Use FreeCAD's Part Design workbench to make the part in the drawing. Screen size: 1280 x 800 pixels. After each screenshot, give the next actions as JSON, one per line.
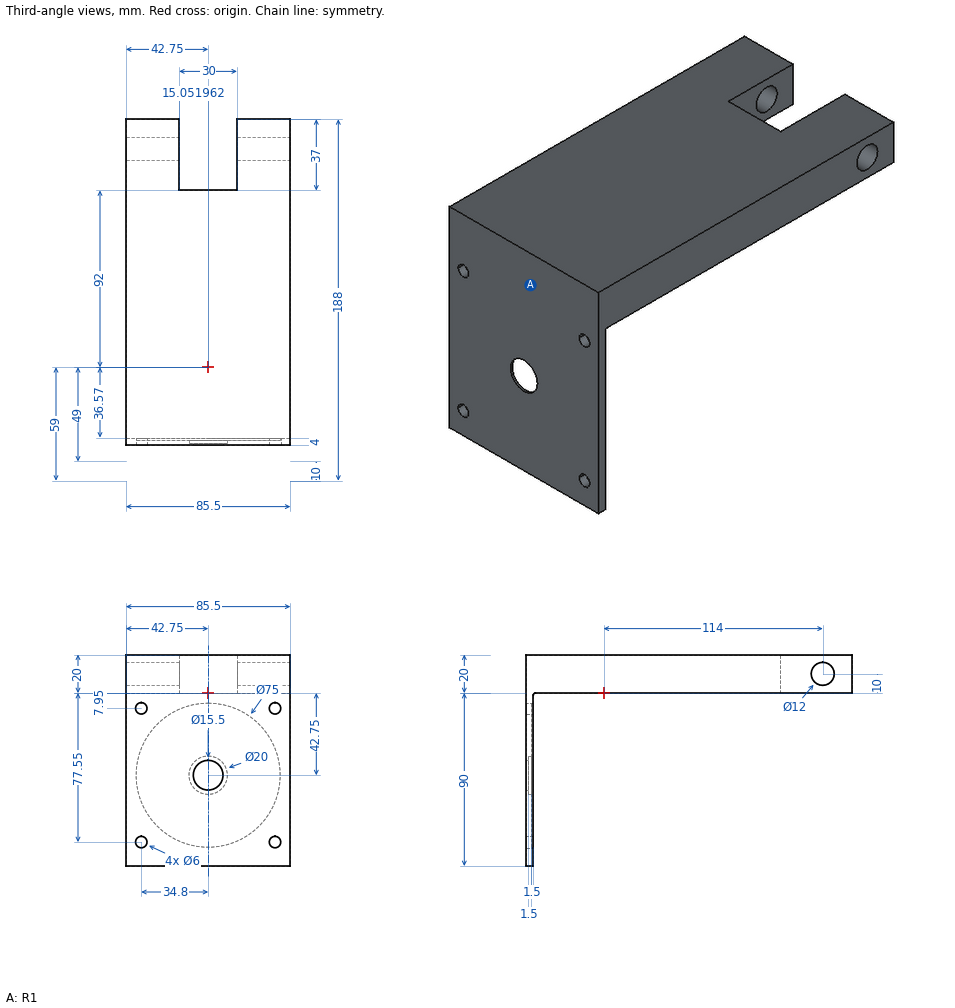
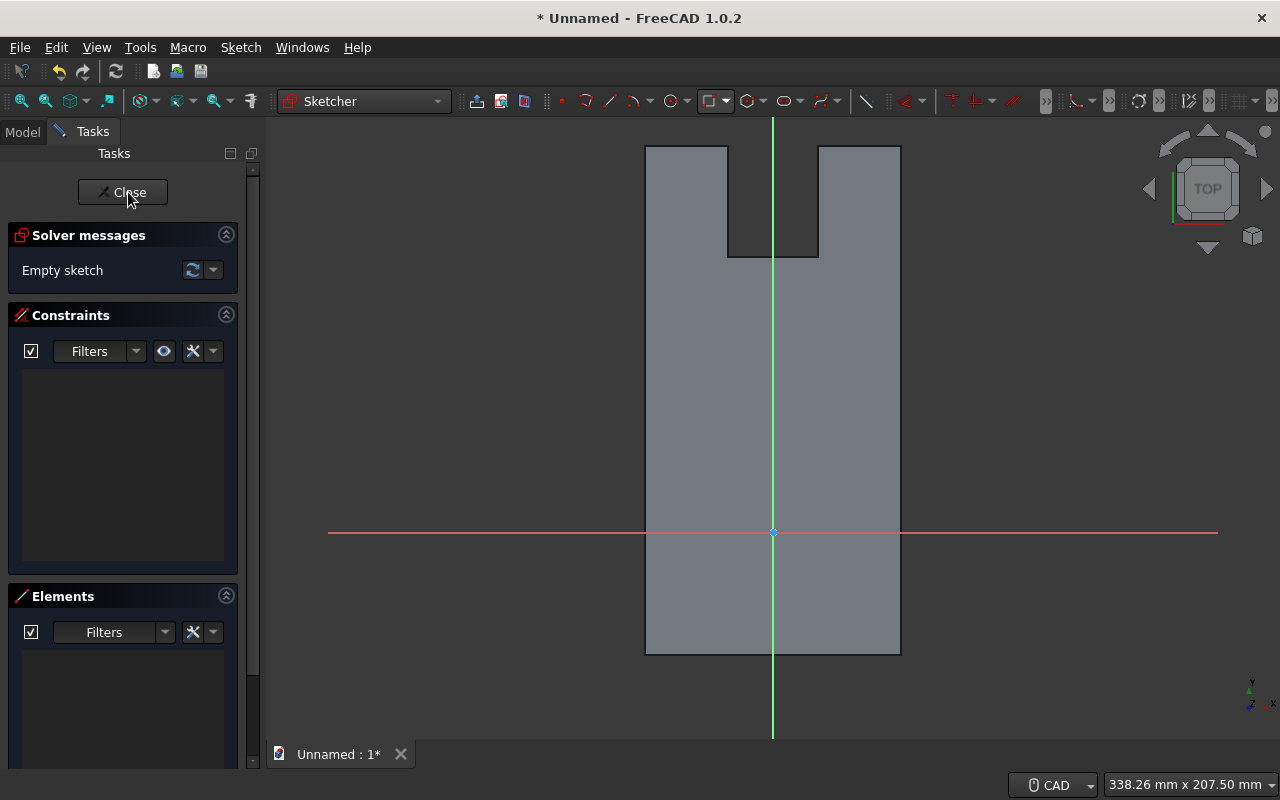
{"action": "scroll", "coordinate": [829, 711], "scroll_direction": "up", "scroll_amount": 4}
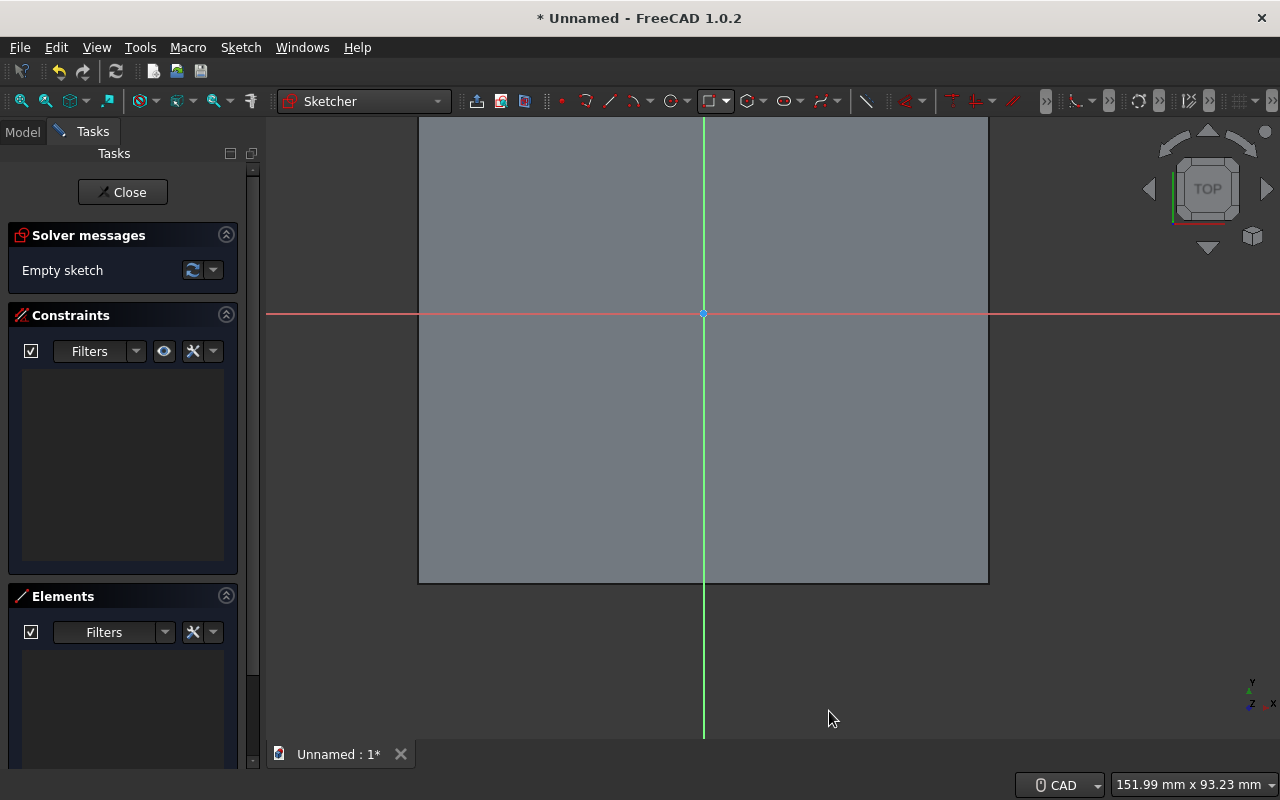
{"action": "key", "text": "g r"}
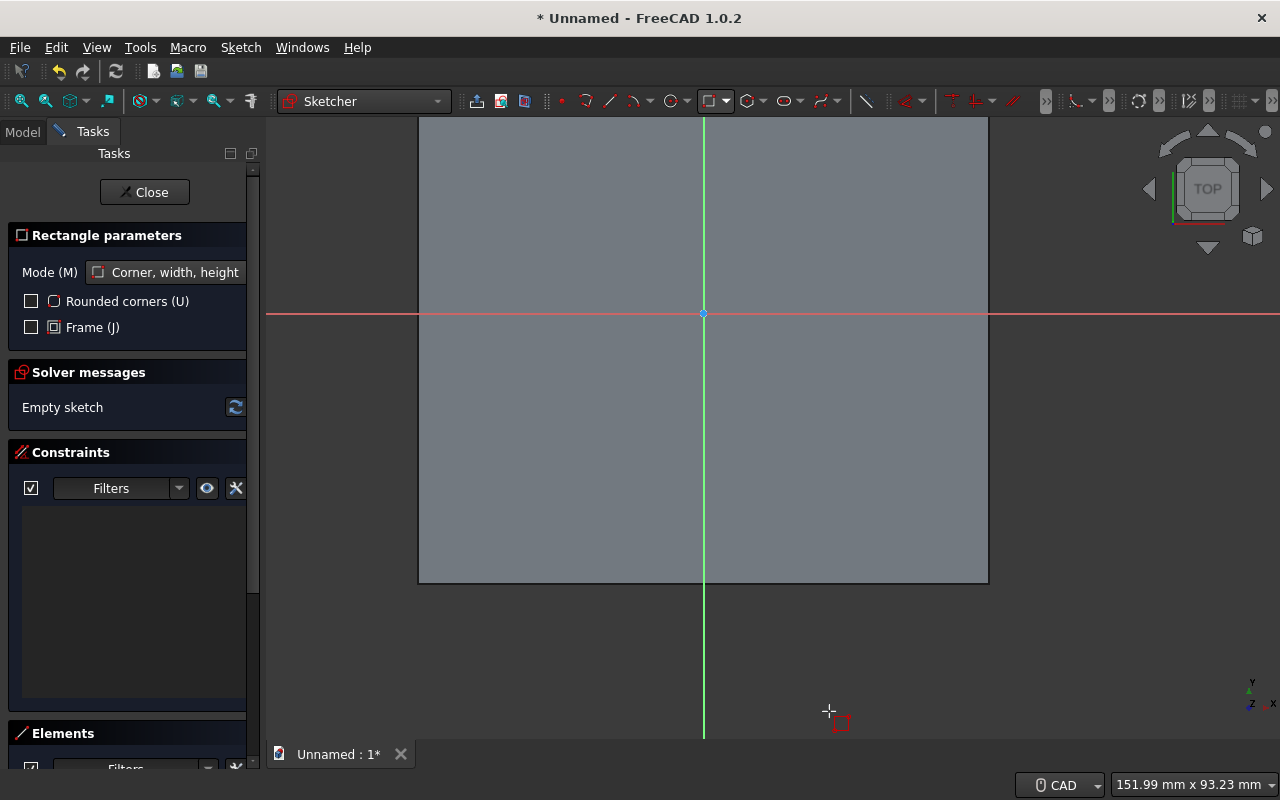
{"action": "left_click", "coordinate": [418, 557]}
{"action": "mouse_move", "coordinate": [989, 584]}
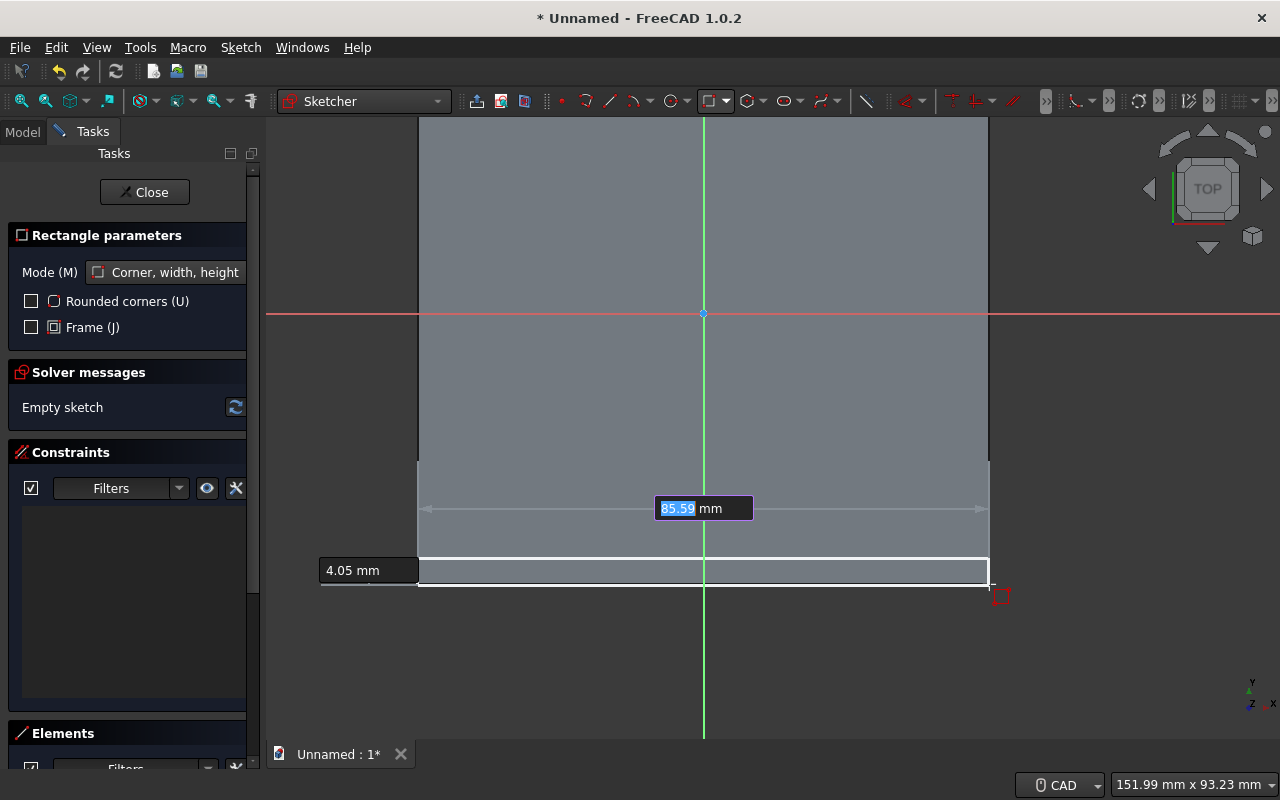
{"action": "type", "text": "85.5"}
{"action": "key", "text": "Tab"}
{"action": "type", "text": "4"}
{"action": "key", "text": "Return"}
{"action": "key", "text": "Escape"}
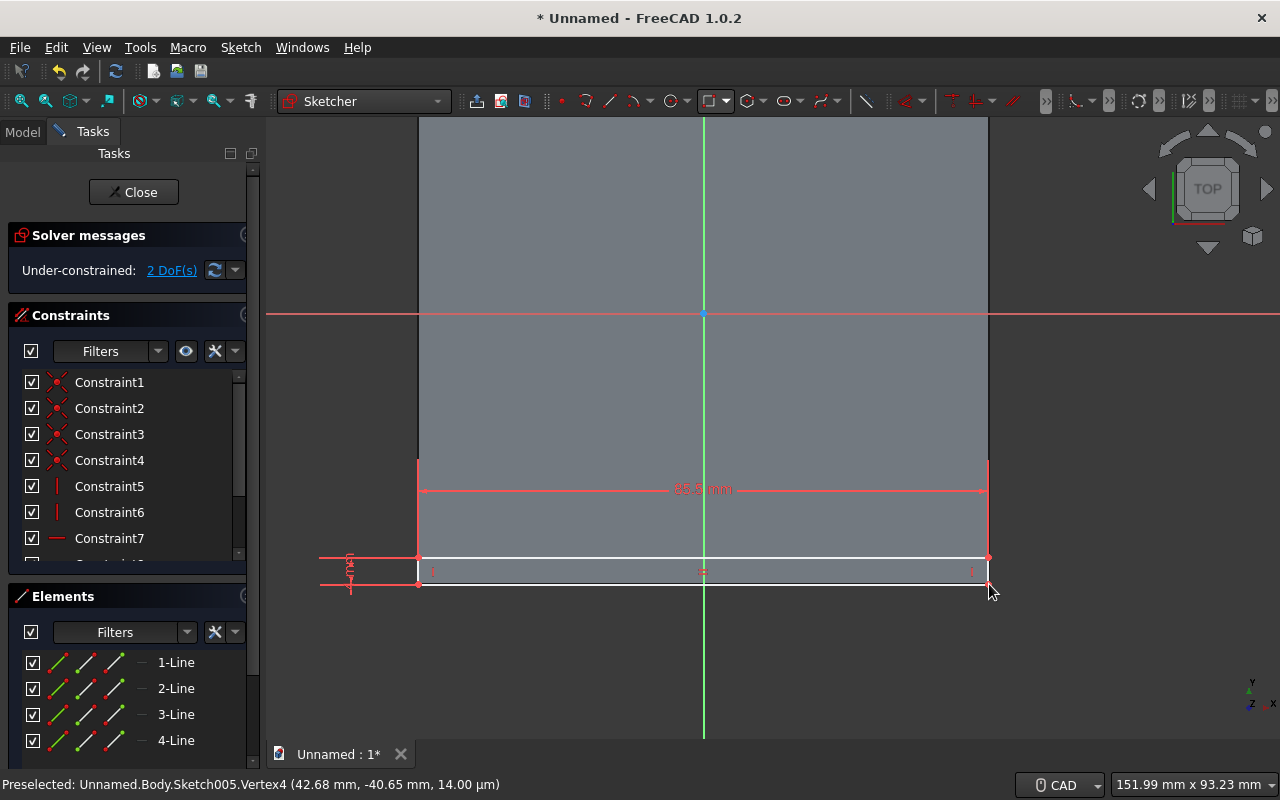
{"action": "key", "text": "d"}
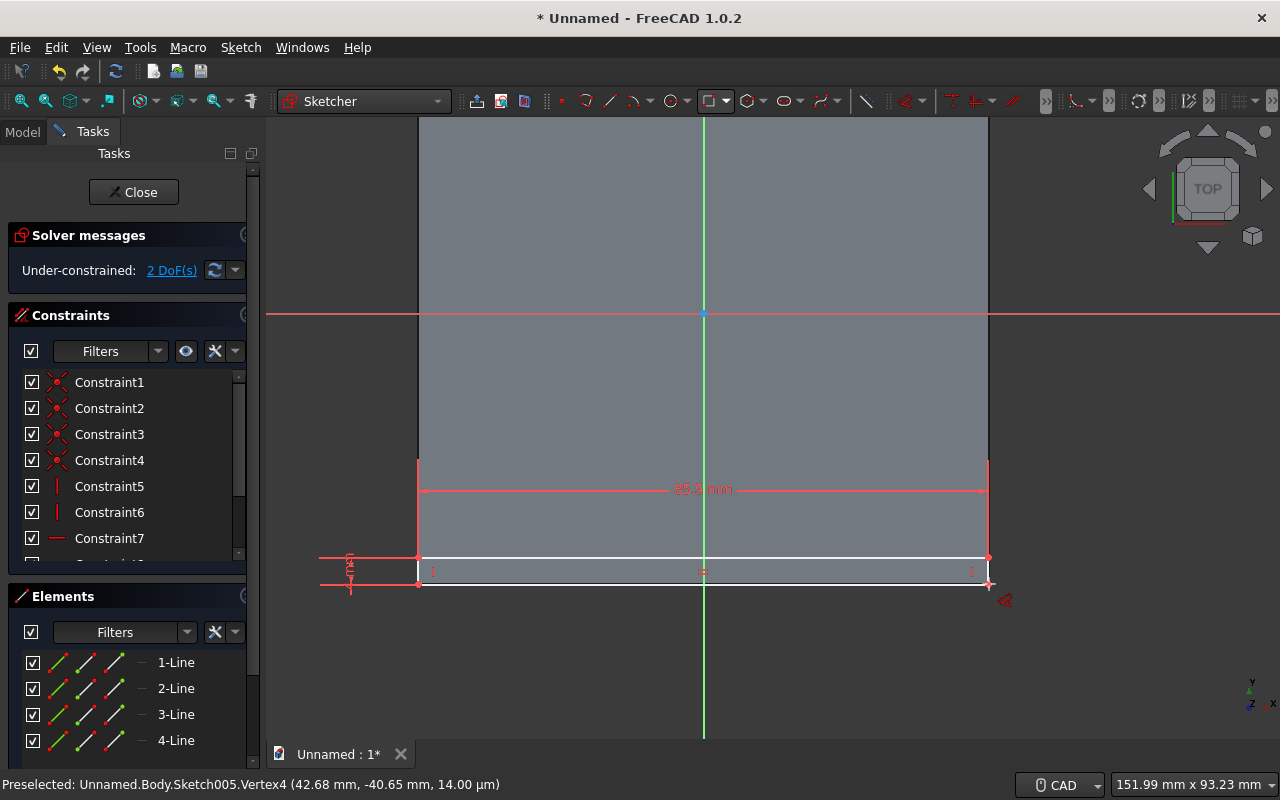
{"action": "left_click", "coordinate": [418, 558]}
{"action": "left_click", "coordinate": [561, 279]}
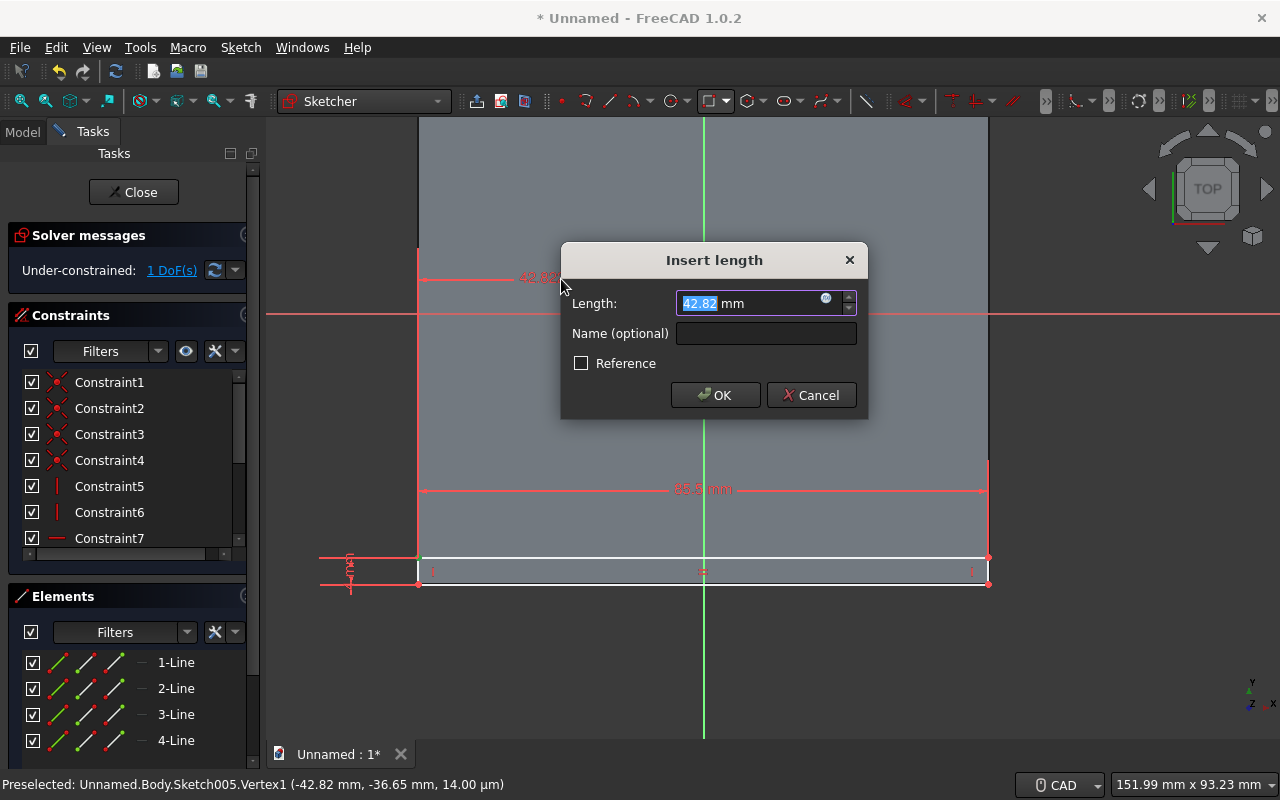
{"action": "type", "text": "42.75"}
{"action": "key", "text": "Return"}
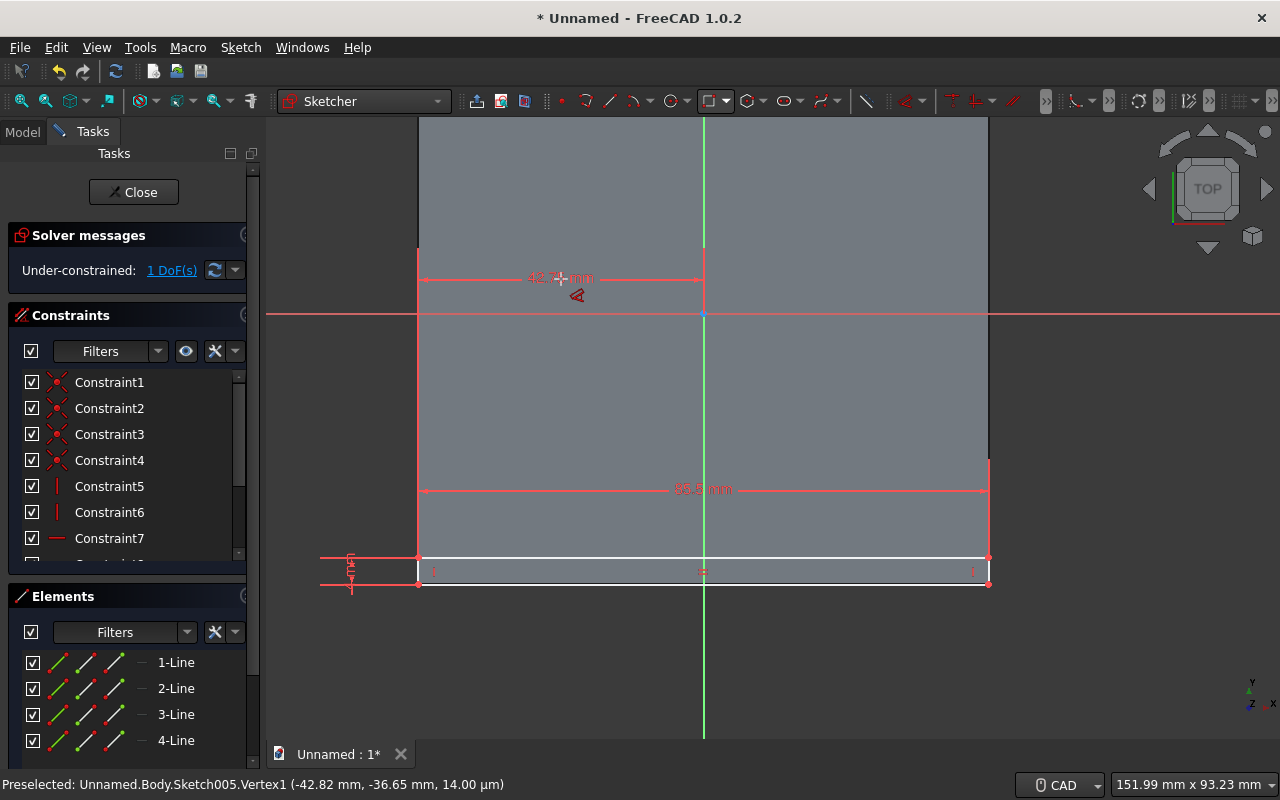
{"action": "left_click", "coordinate": [418, 558]}
{"action": "left_click", "coordinate": [384, 436]}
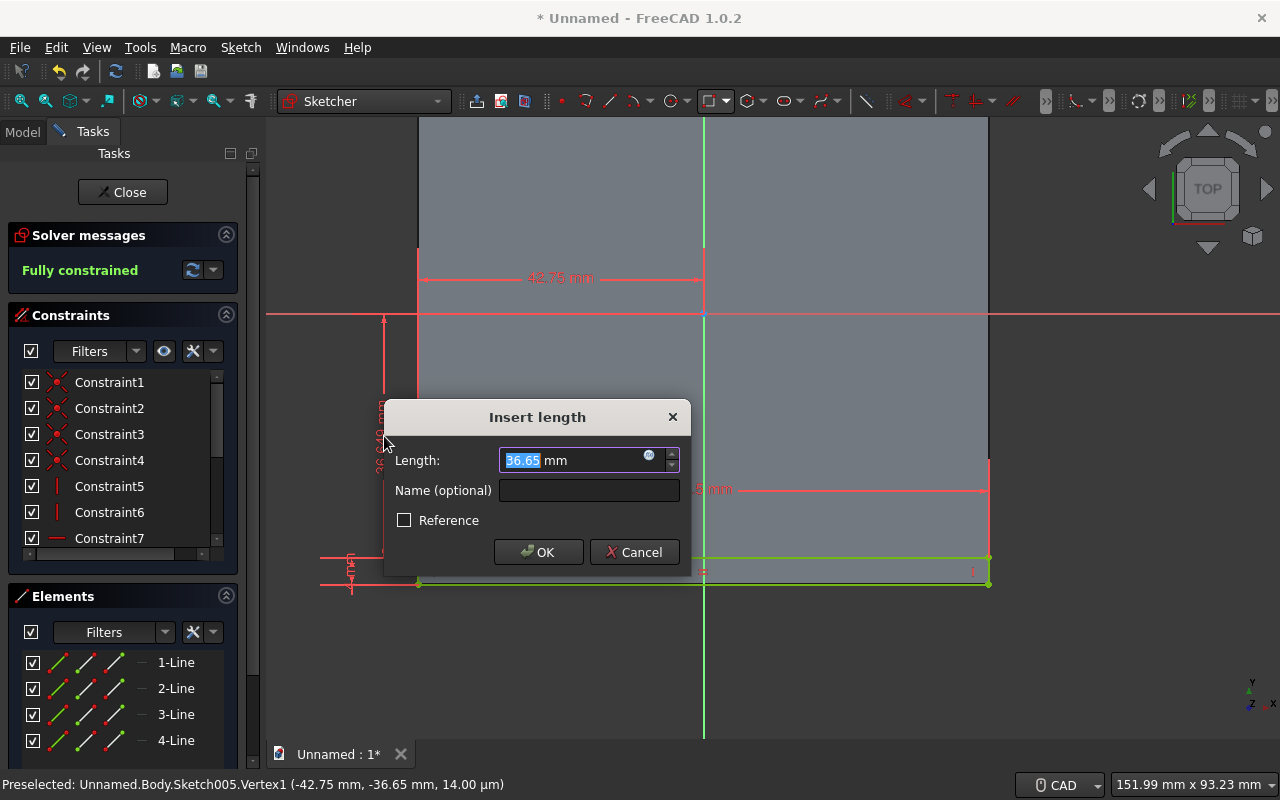
{"action": "type", "text": "36.57"}
{"action": "key", "text": "Return"}
{"action": "key", "text": "Escape"}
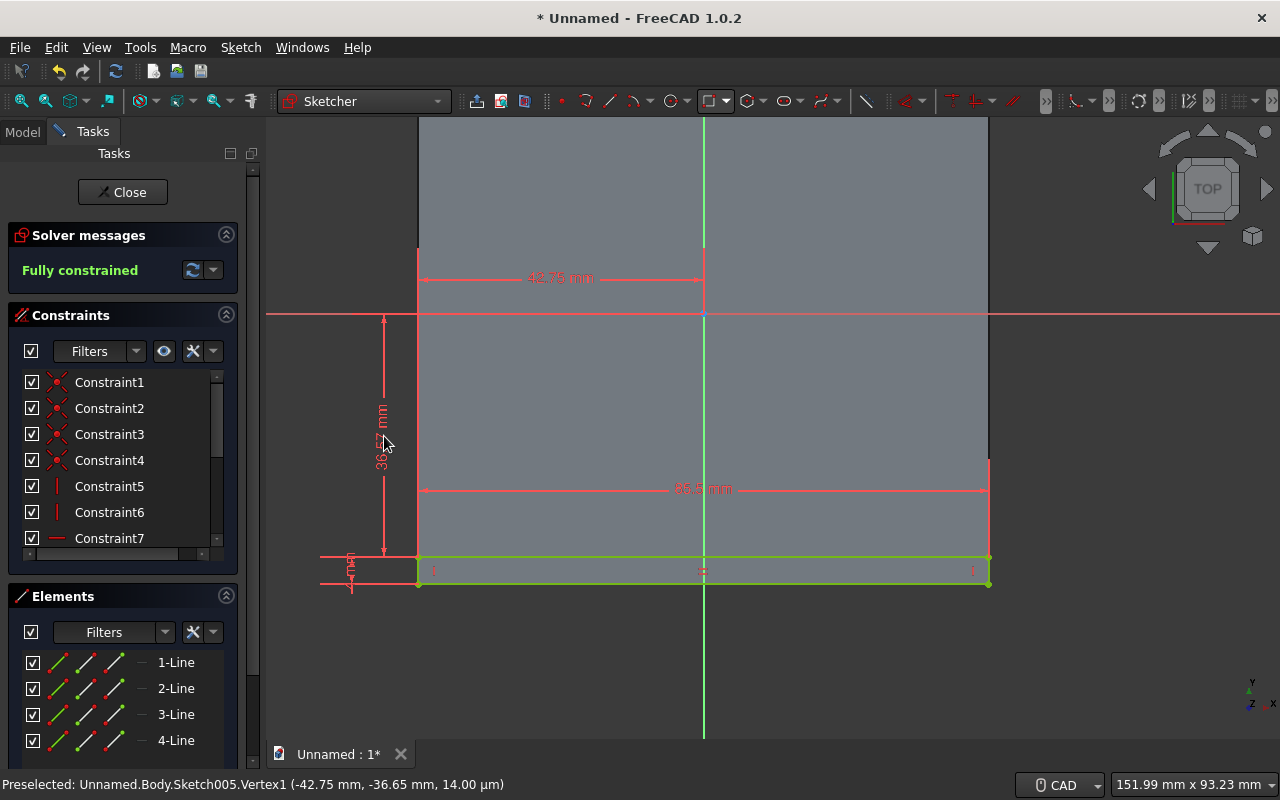
{"action": "left_click", "coordinate": [123, 192]}